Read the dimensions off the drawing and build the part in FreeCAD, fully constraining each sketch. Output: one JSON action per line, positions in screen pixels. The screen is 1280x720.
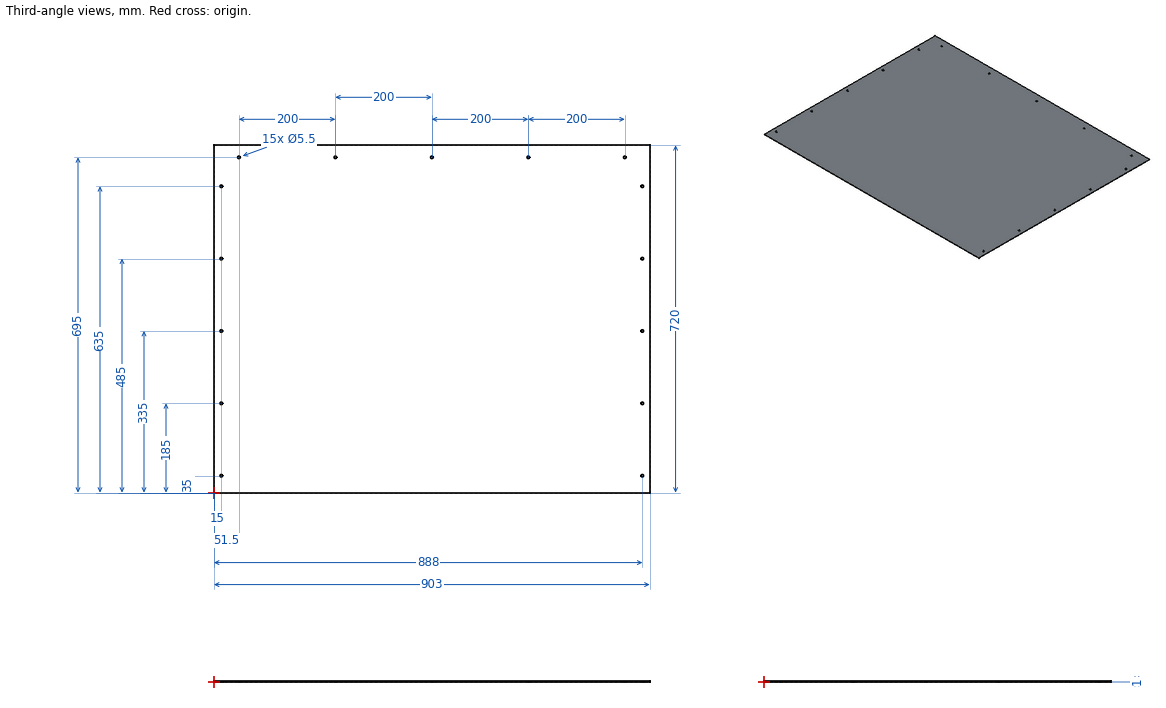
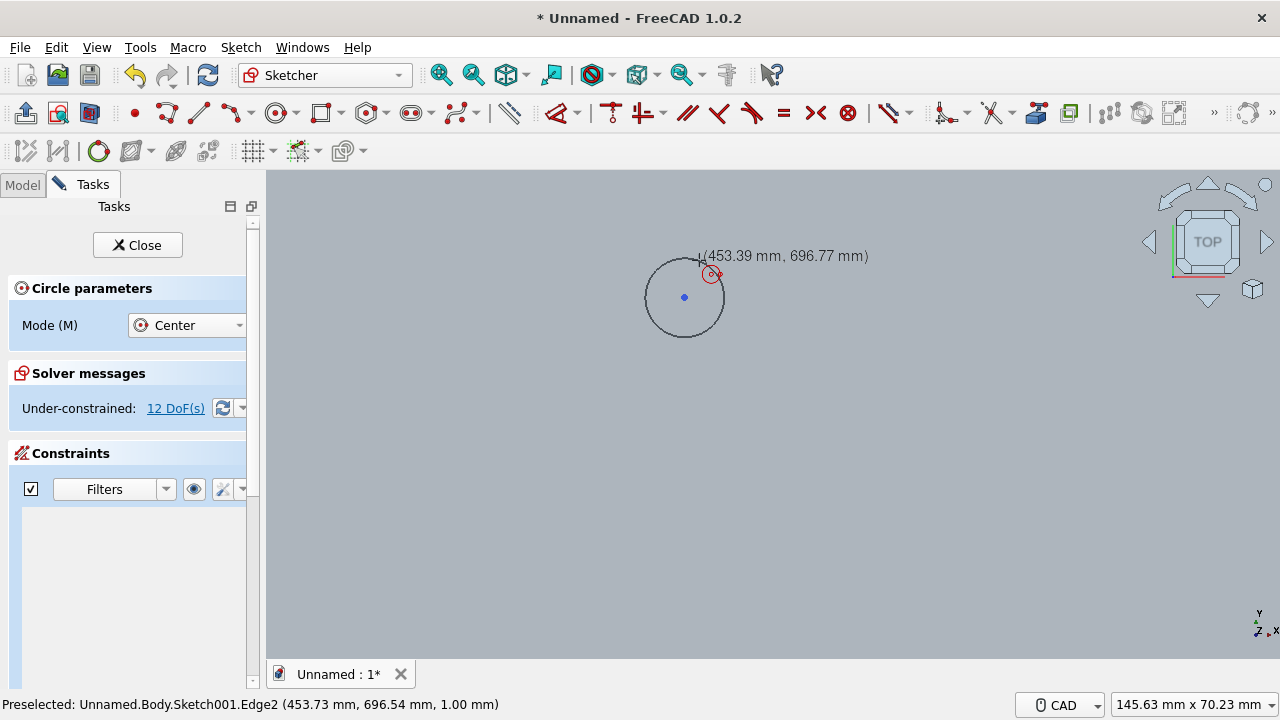
{"action": "scroll", "coordinate": [708, 268], "scroll_direction": "down", "scroll_amount": 14}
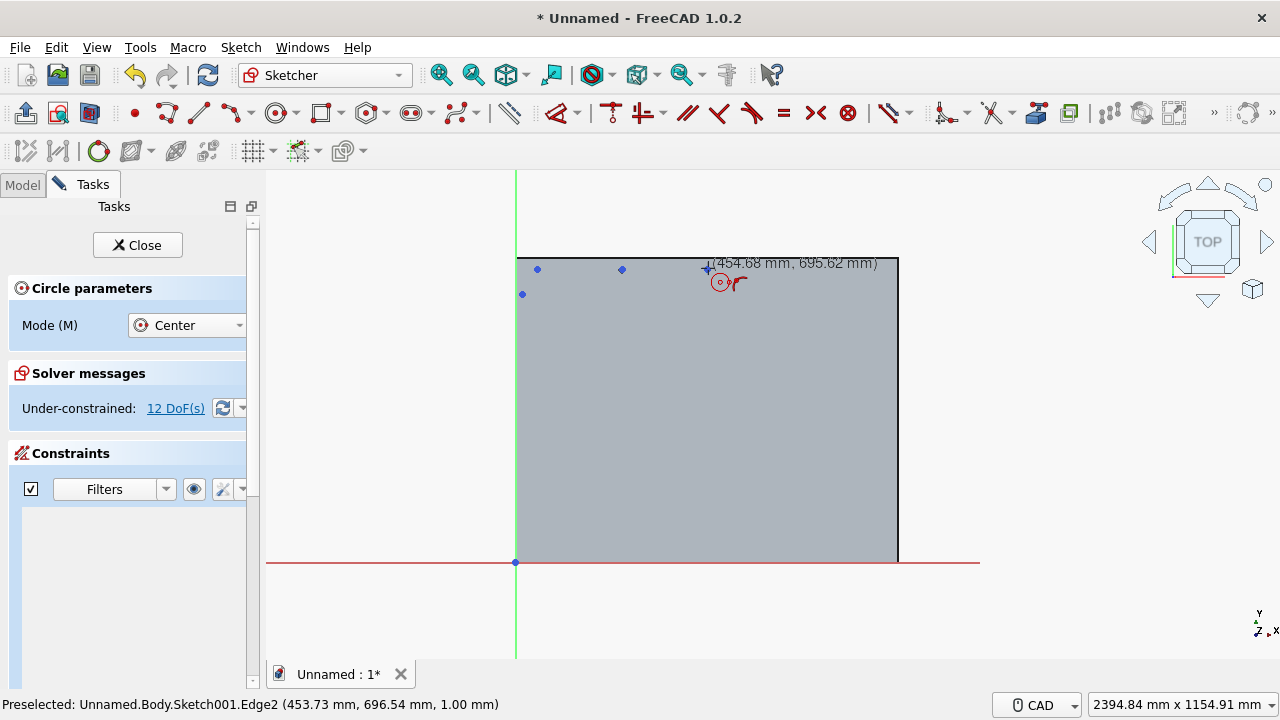
{"action": "scroll", "coordinate": [792, 269], "scroll_direction": "up", "scroll_amount": 15}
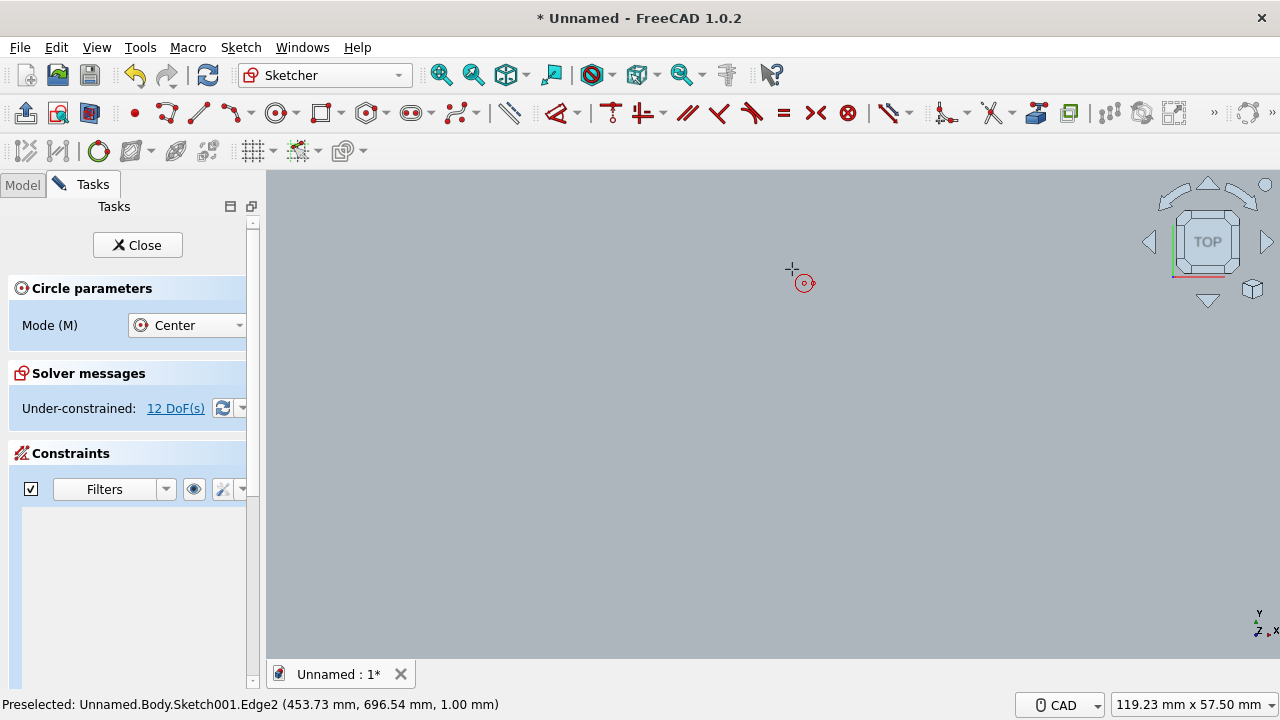
{"action": "scroll", "coordinate": [793, 269], "scroll_direction": "down", "scroll_amount": 15}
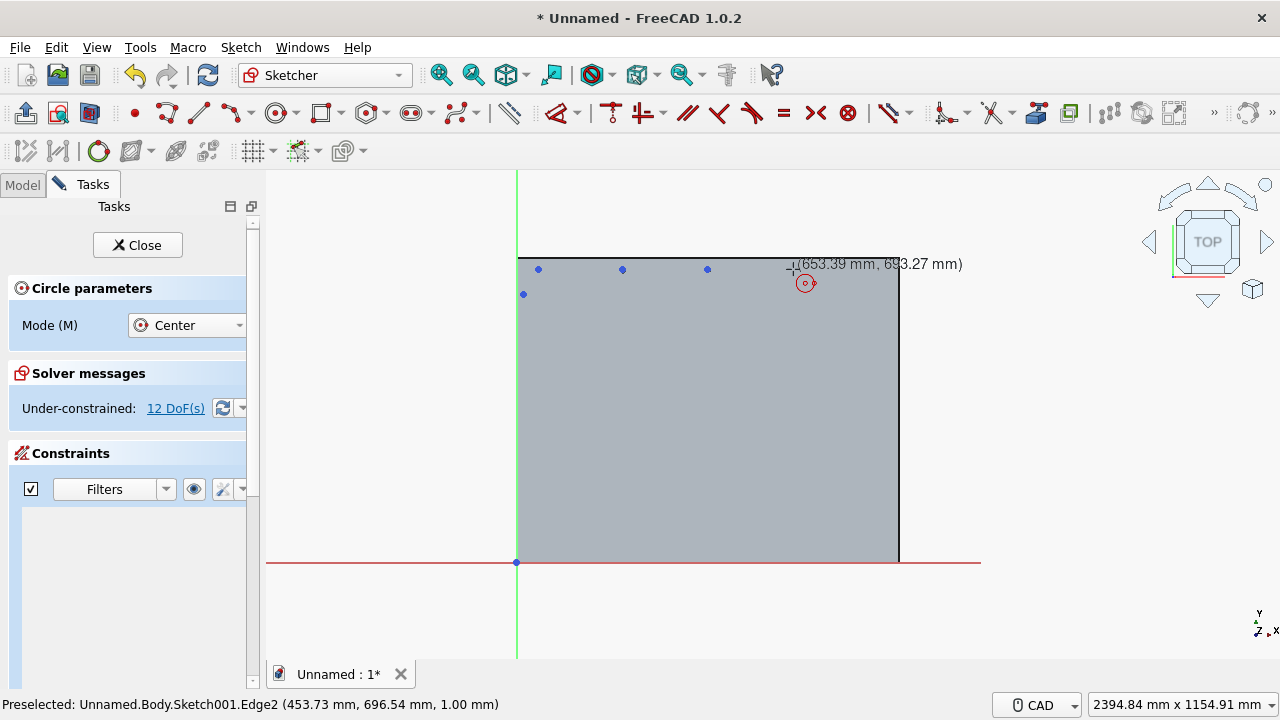
{"action": "left_click", "coordinate": [793, 269]}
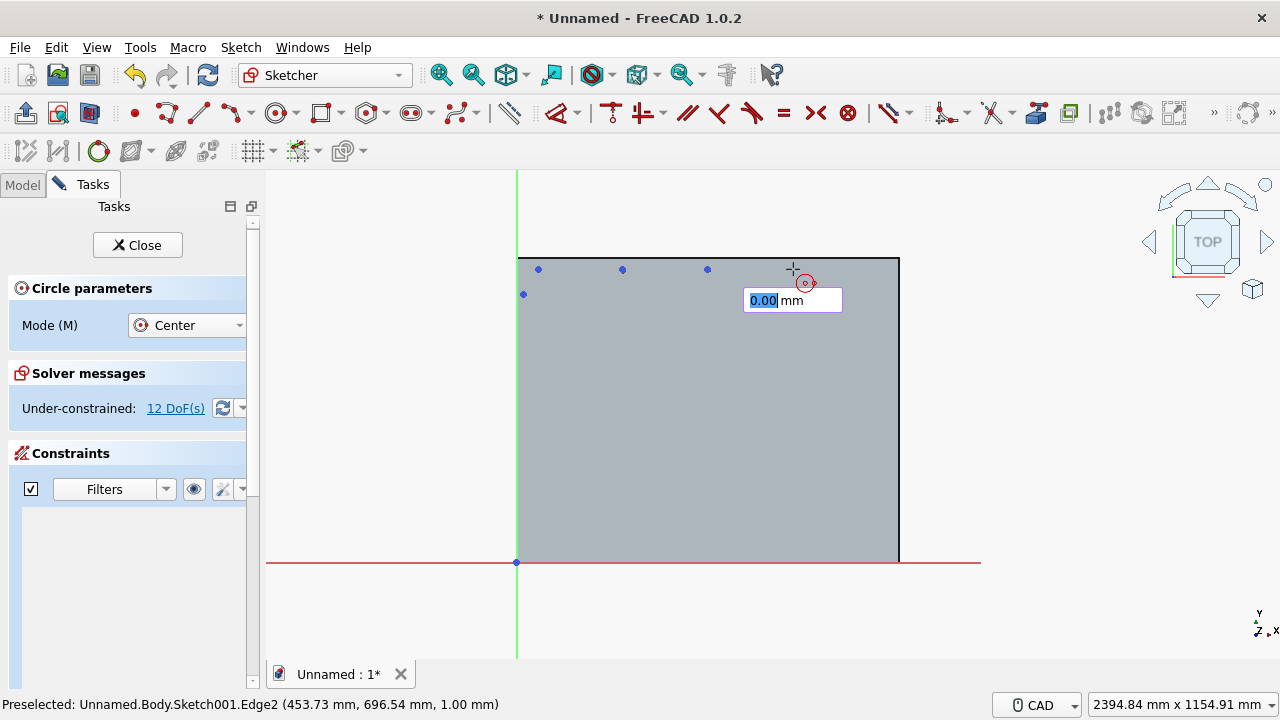
{"action": "scroll", "coordinate": [794, 268], "scroll_direction": "up", "scroll_amount": 14}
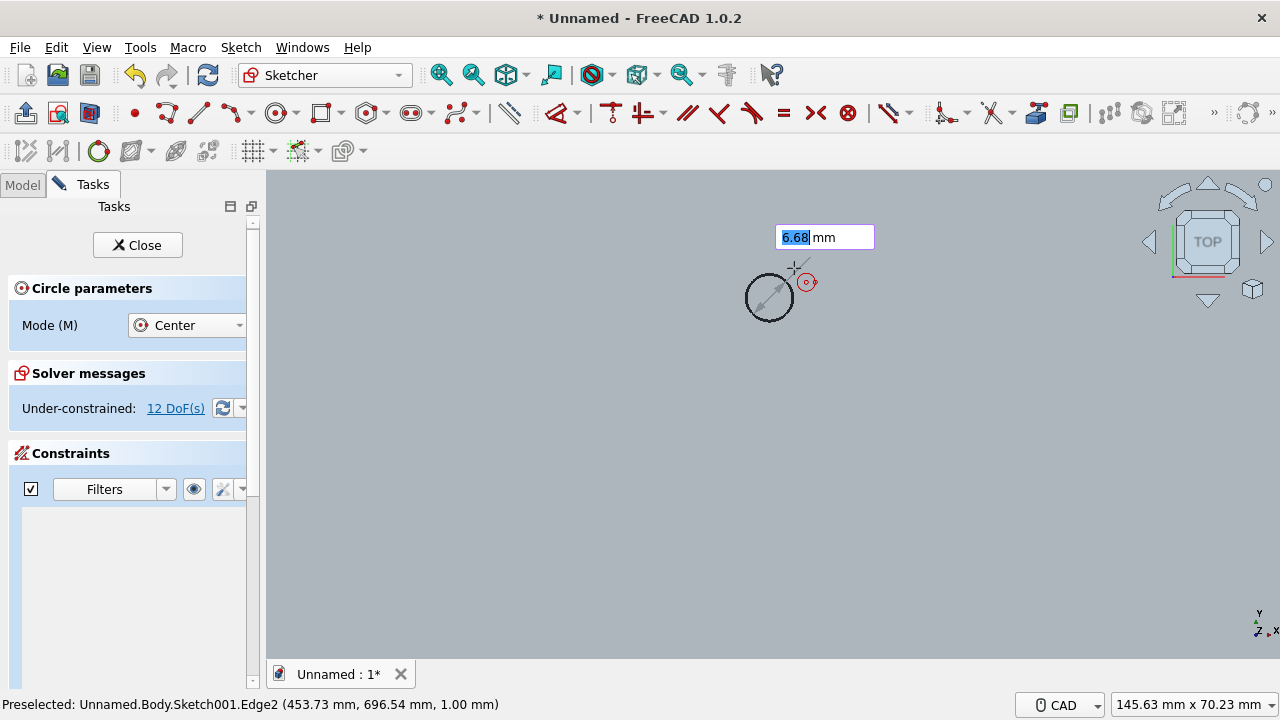
{"action": "left_click", "coordinate": [778, 260]}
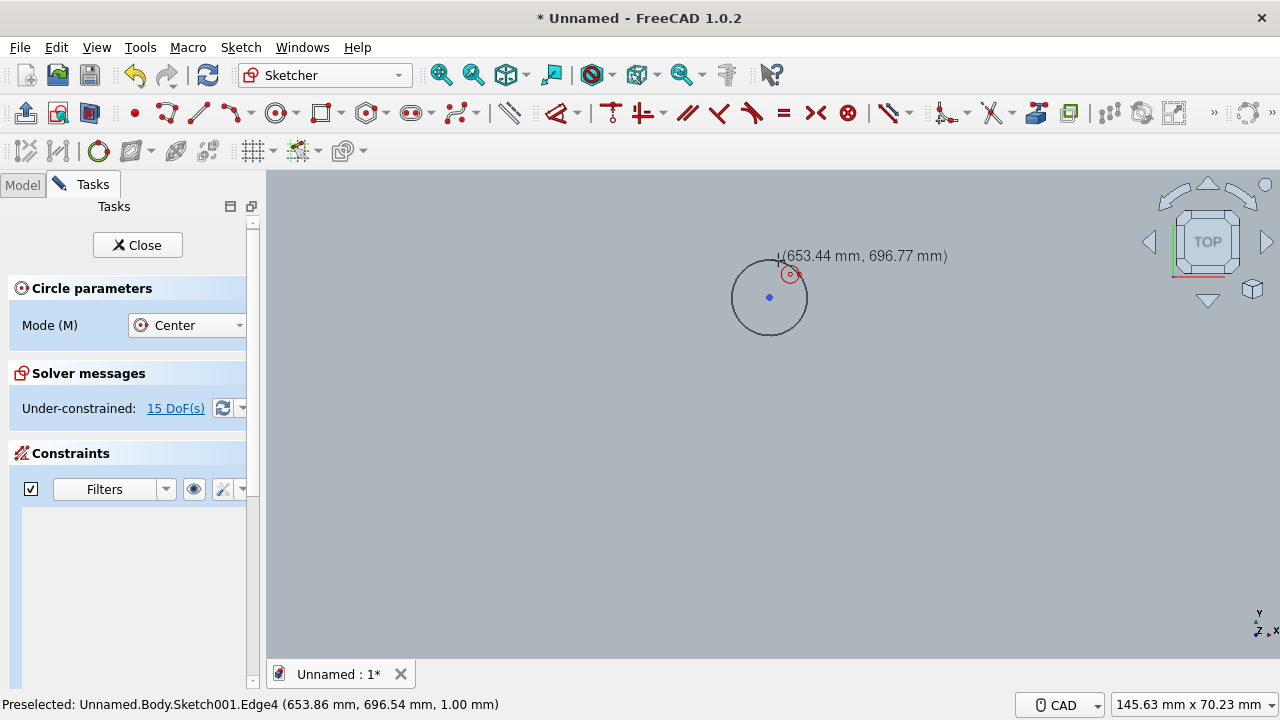
{"action": "scroll", "coordinate": [794, 268], "scroll_direction": "down", "scroll_amount": 14}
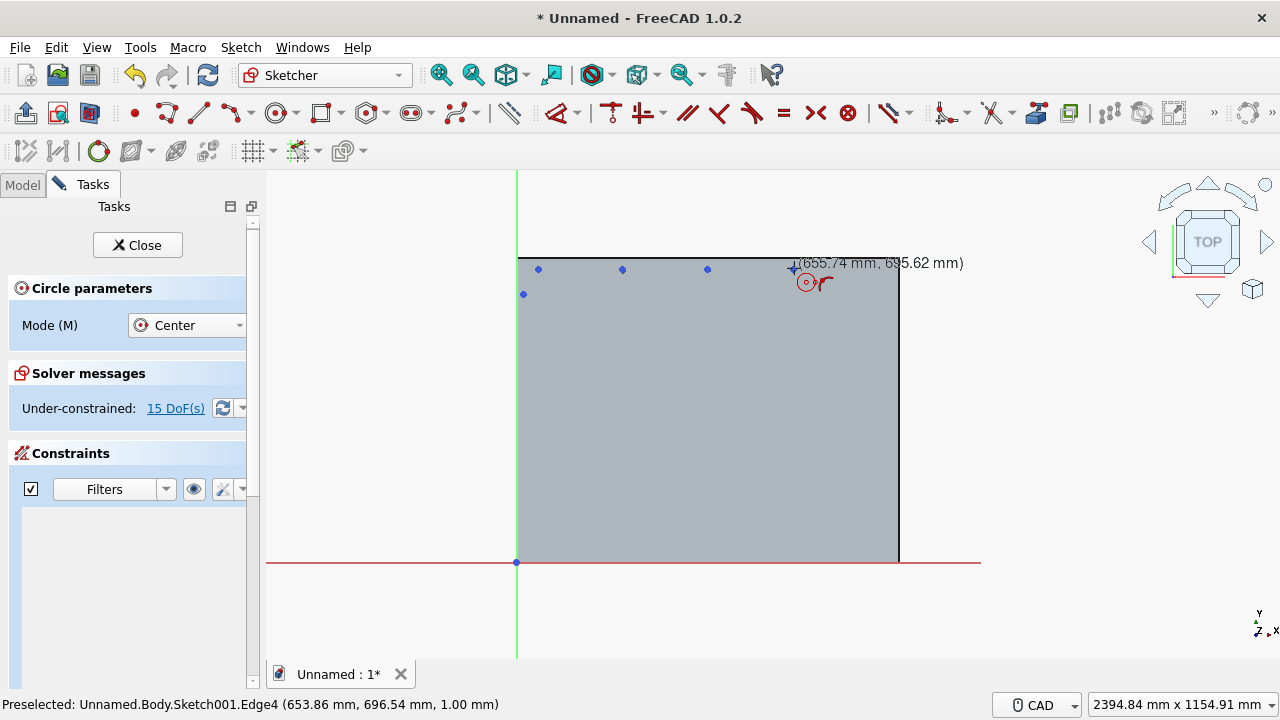
{"action": "scroll", "coordinate": [877, 269], "scroll_direction": "up", "scroll_amount": 15}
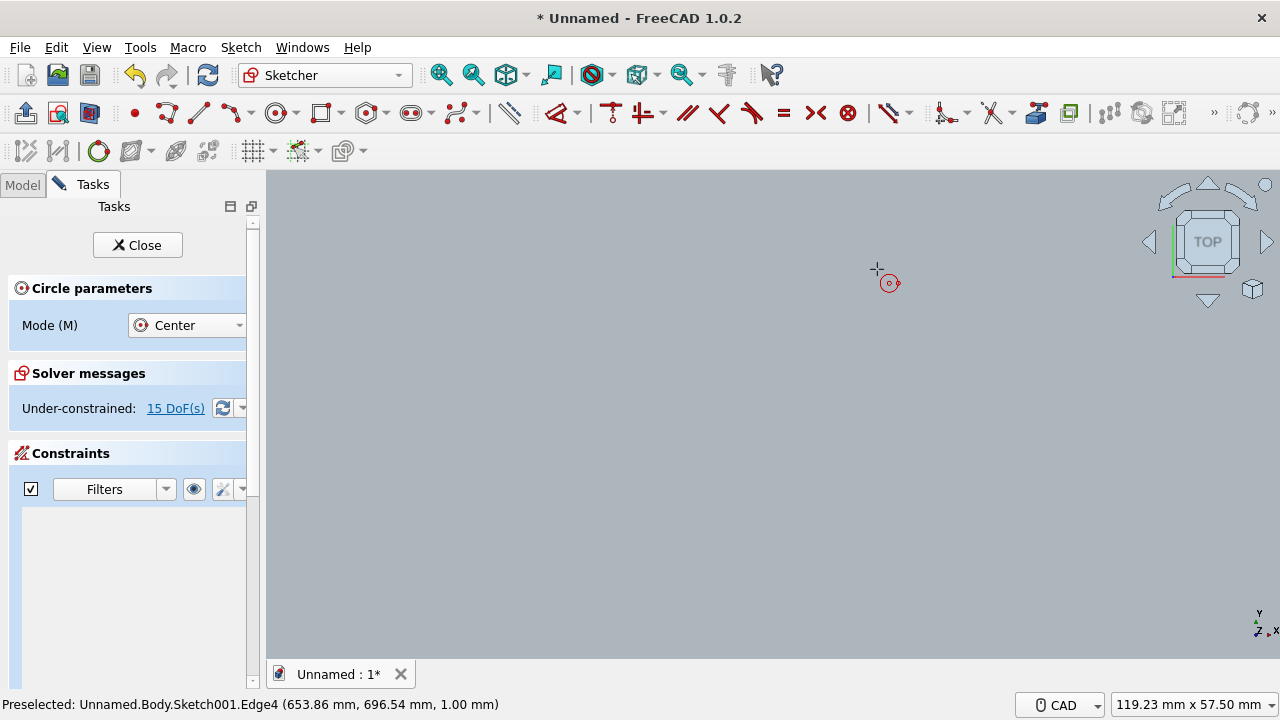
{"action": "scroll", "coordinate": [877, 269], "scroll_direction": "down", "scroll_amount": 15}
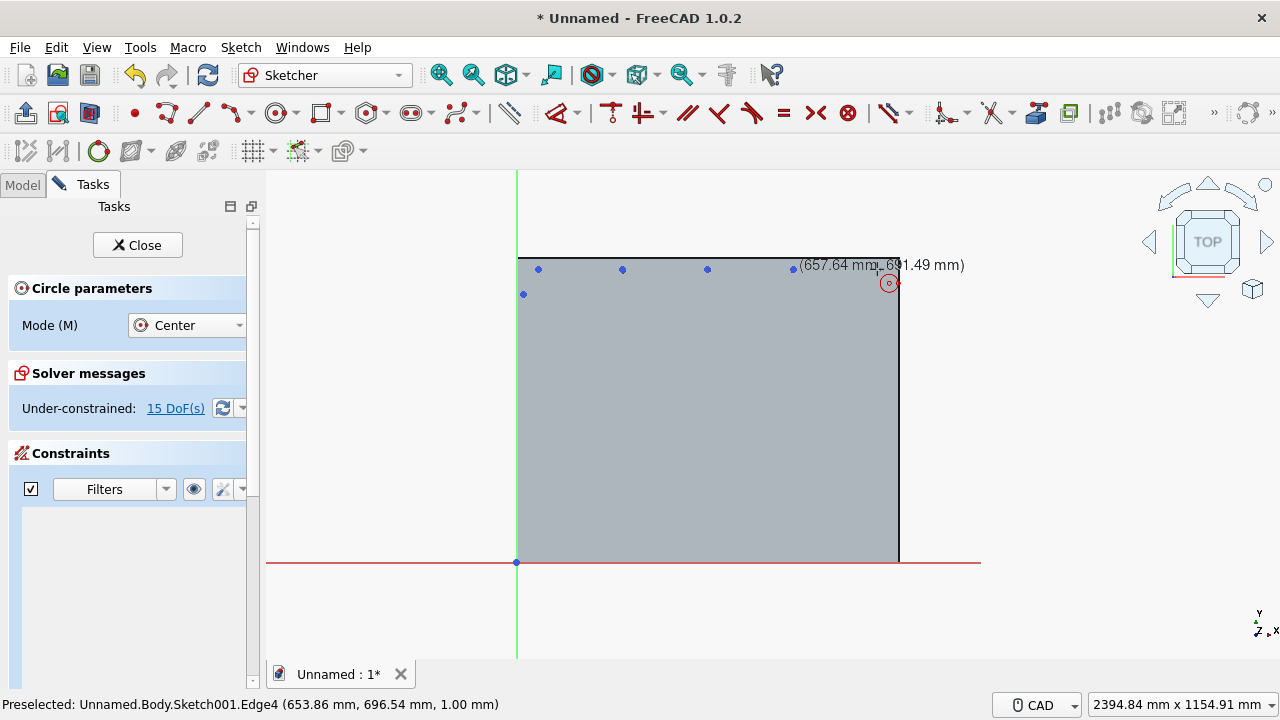
{"action": "left_click", "coordinate": [877, 269]}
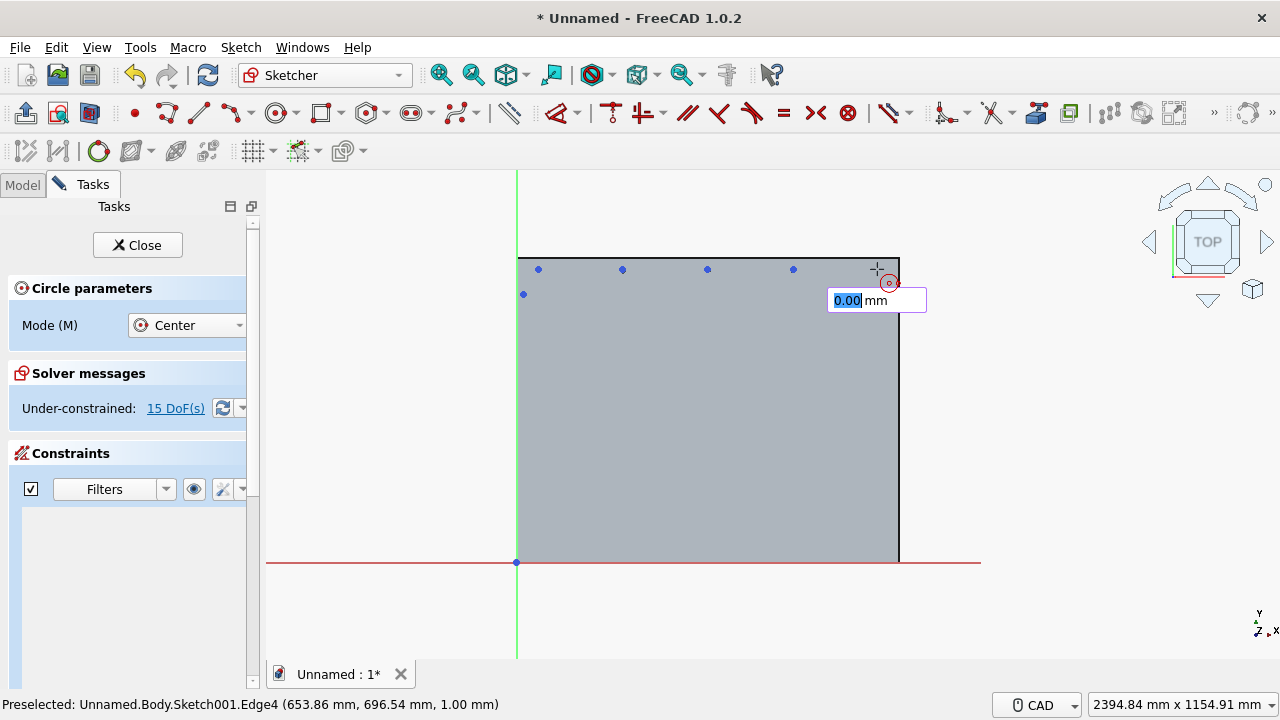
{"action": "scroll", "coordinate": [878, 268], "scroll_direction": "up", "scroll_amount": 14}